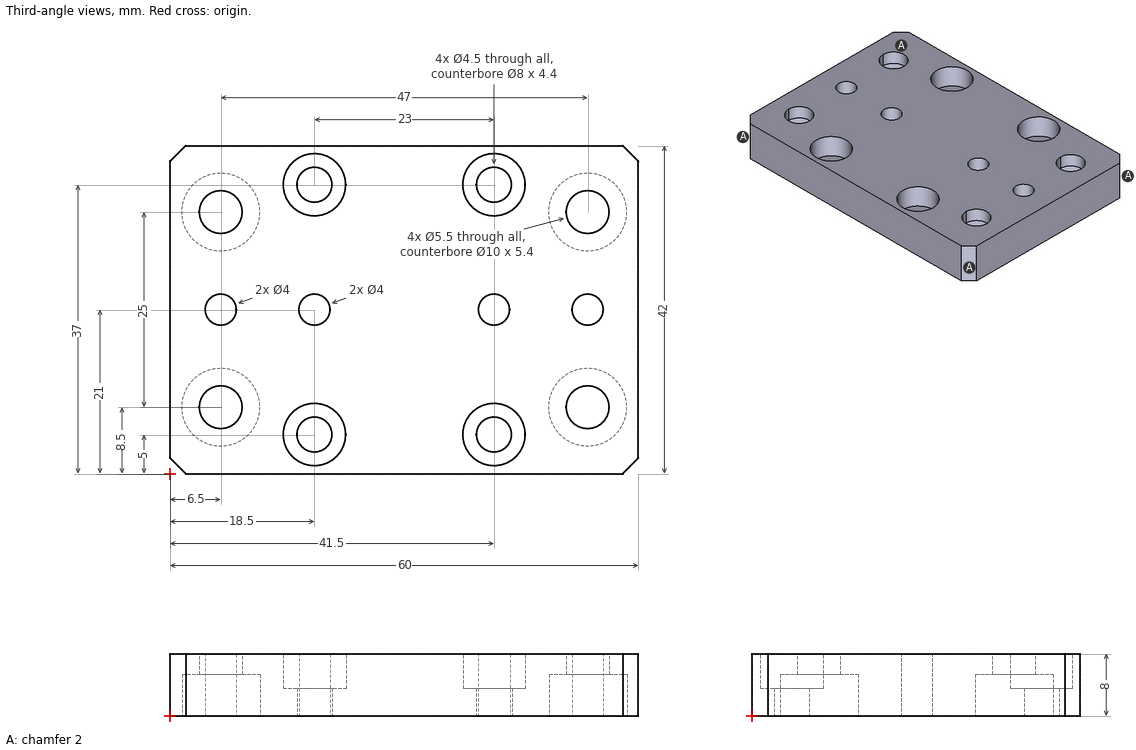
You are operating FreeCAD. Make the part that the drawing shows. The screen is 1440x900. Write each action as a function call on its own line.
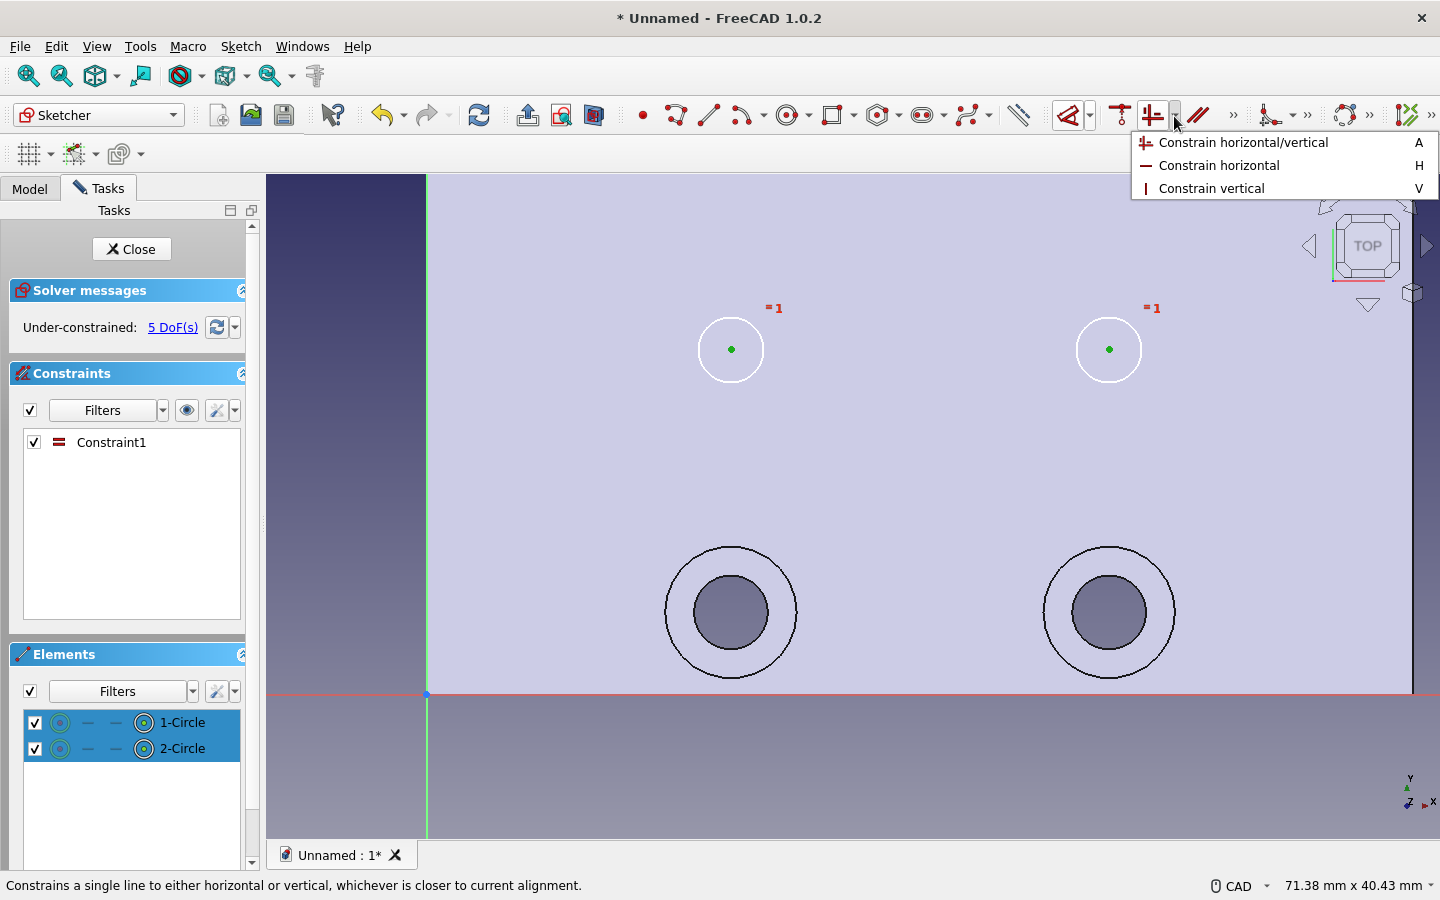
click(1285, 166)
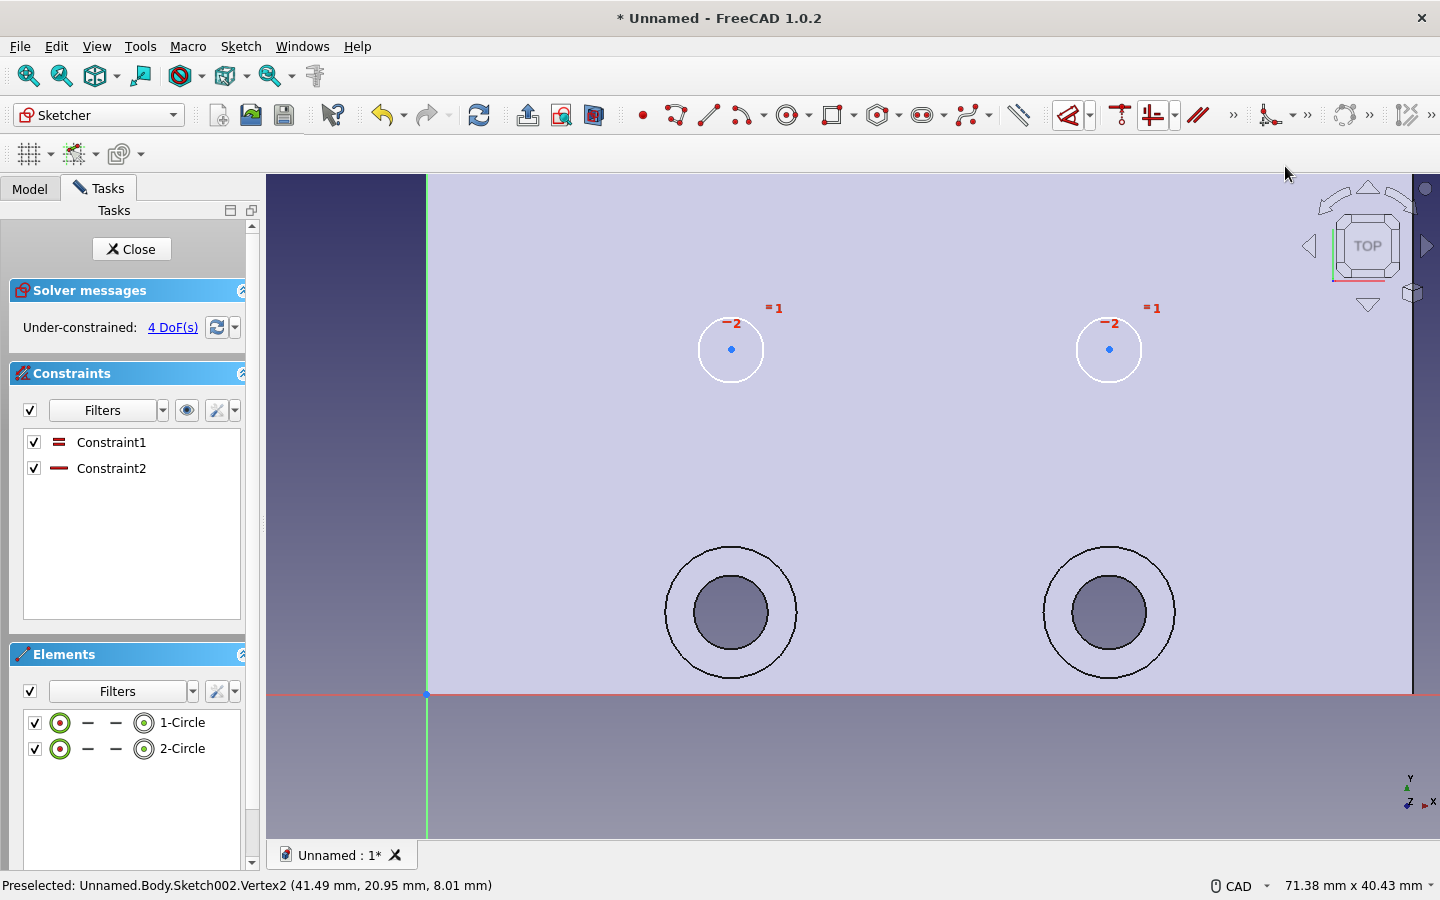
click(754, 327)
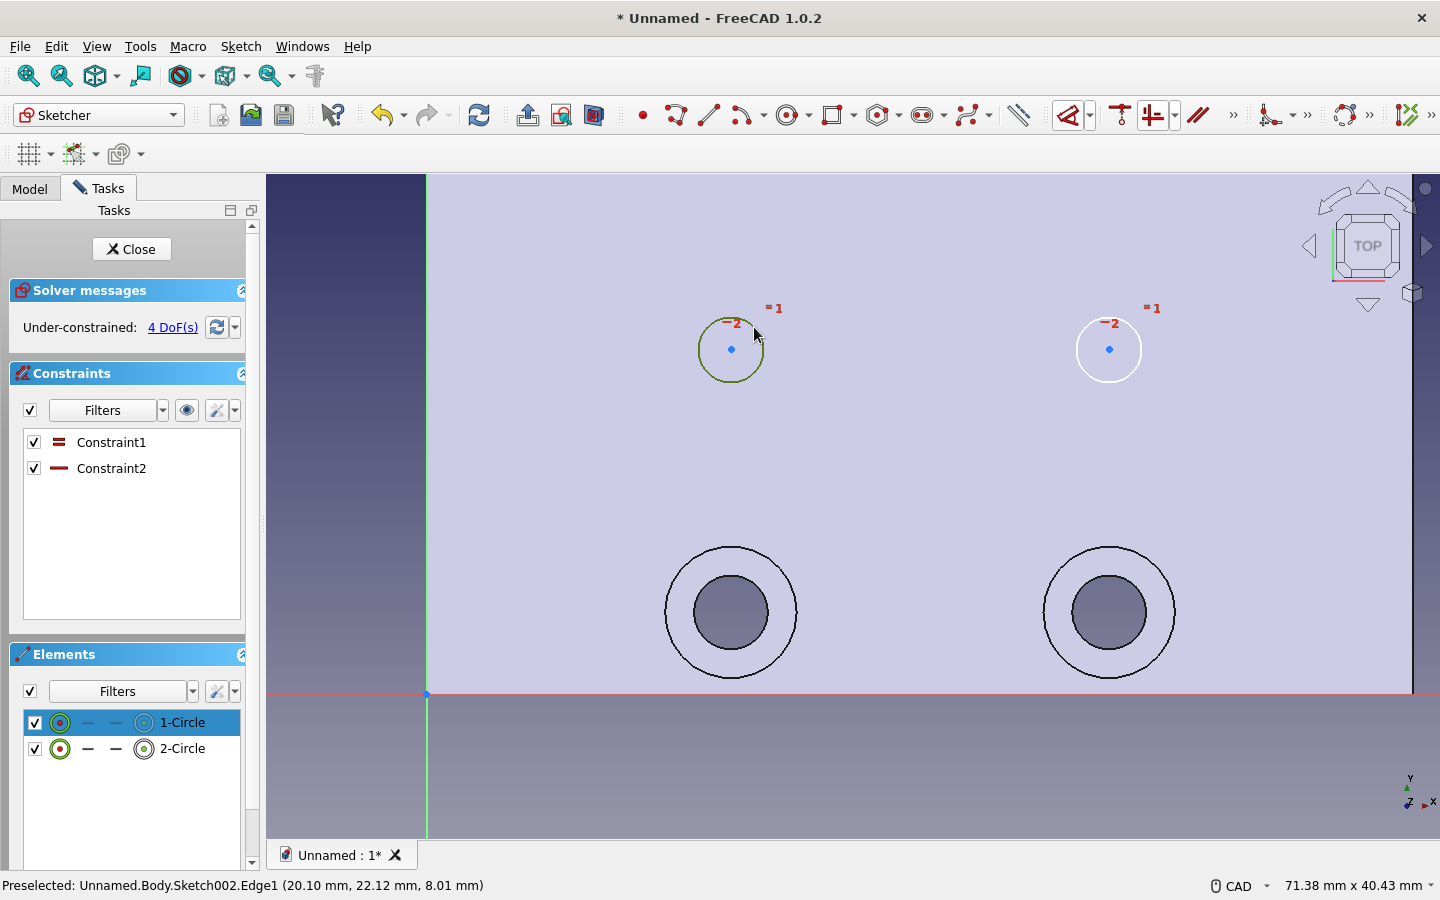
key(k)
key(o)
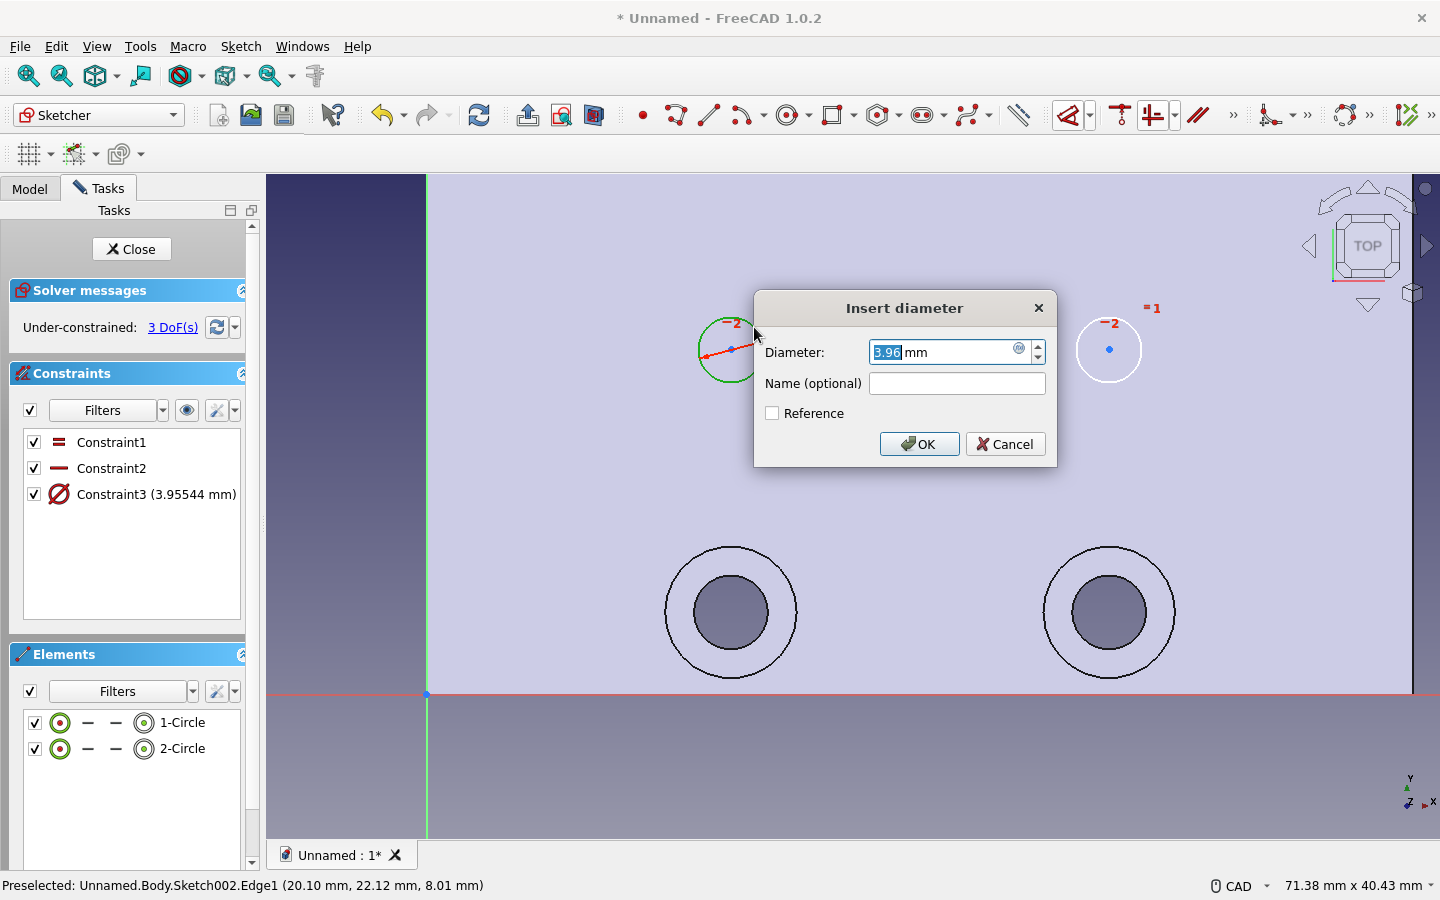
text(4)
key(Return)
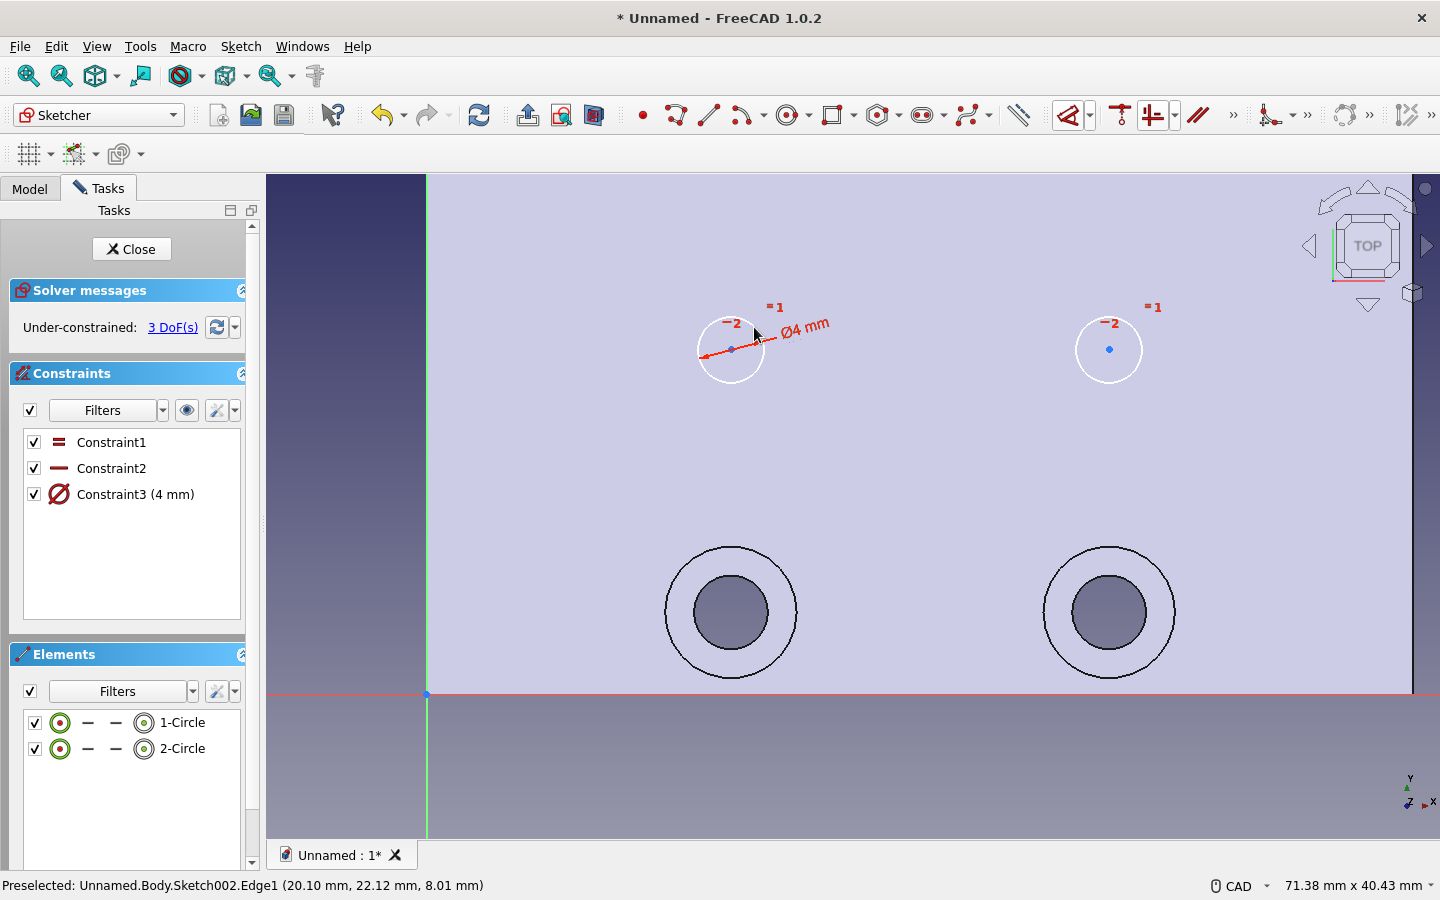
click(731, 350)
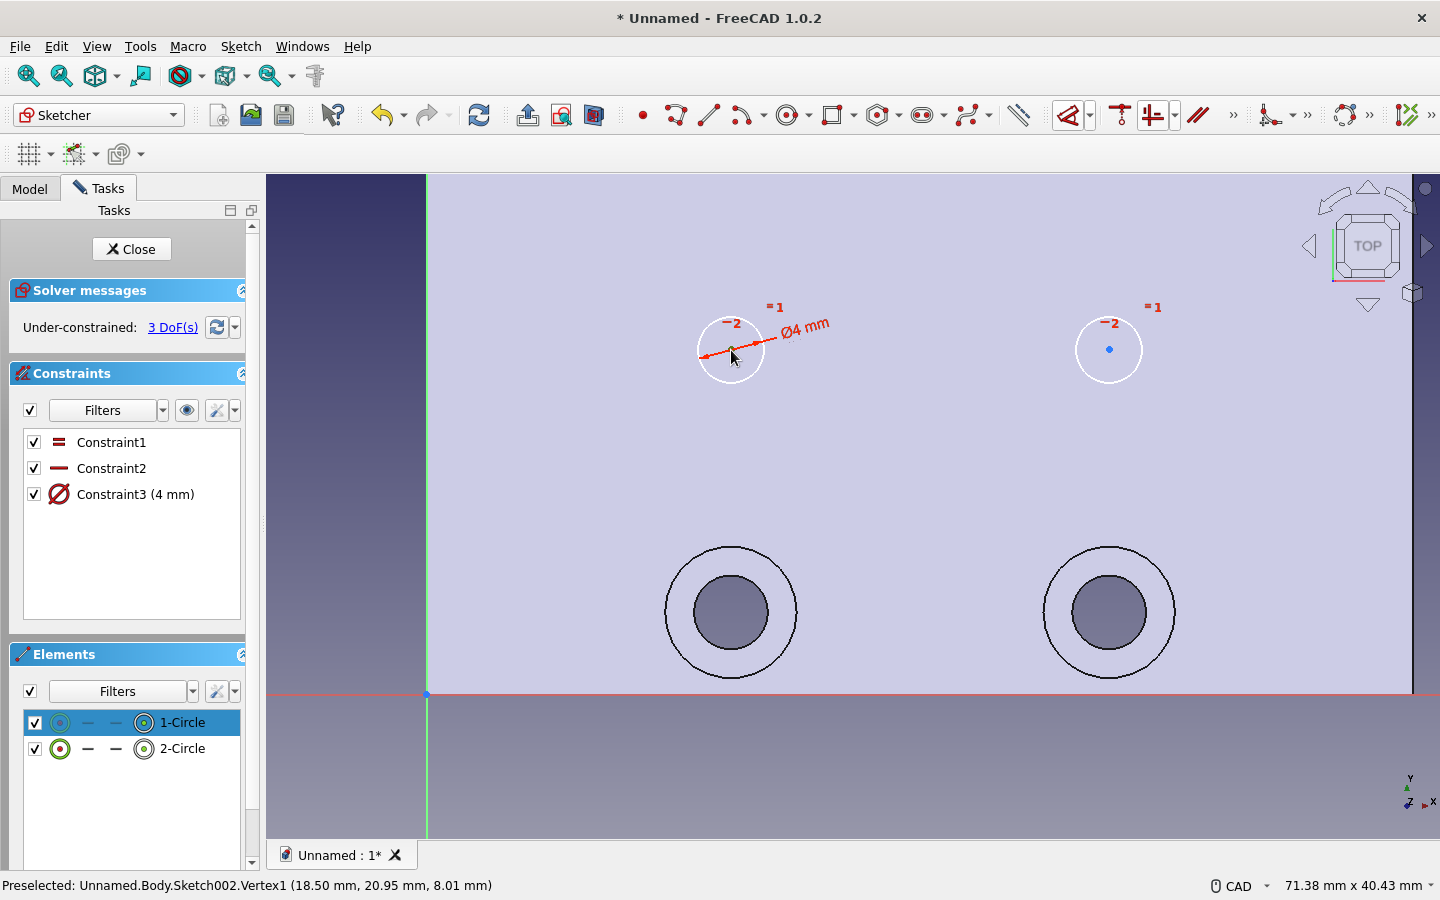
click(1090, 116)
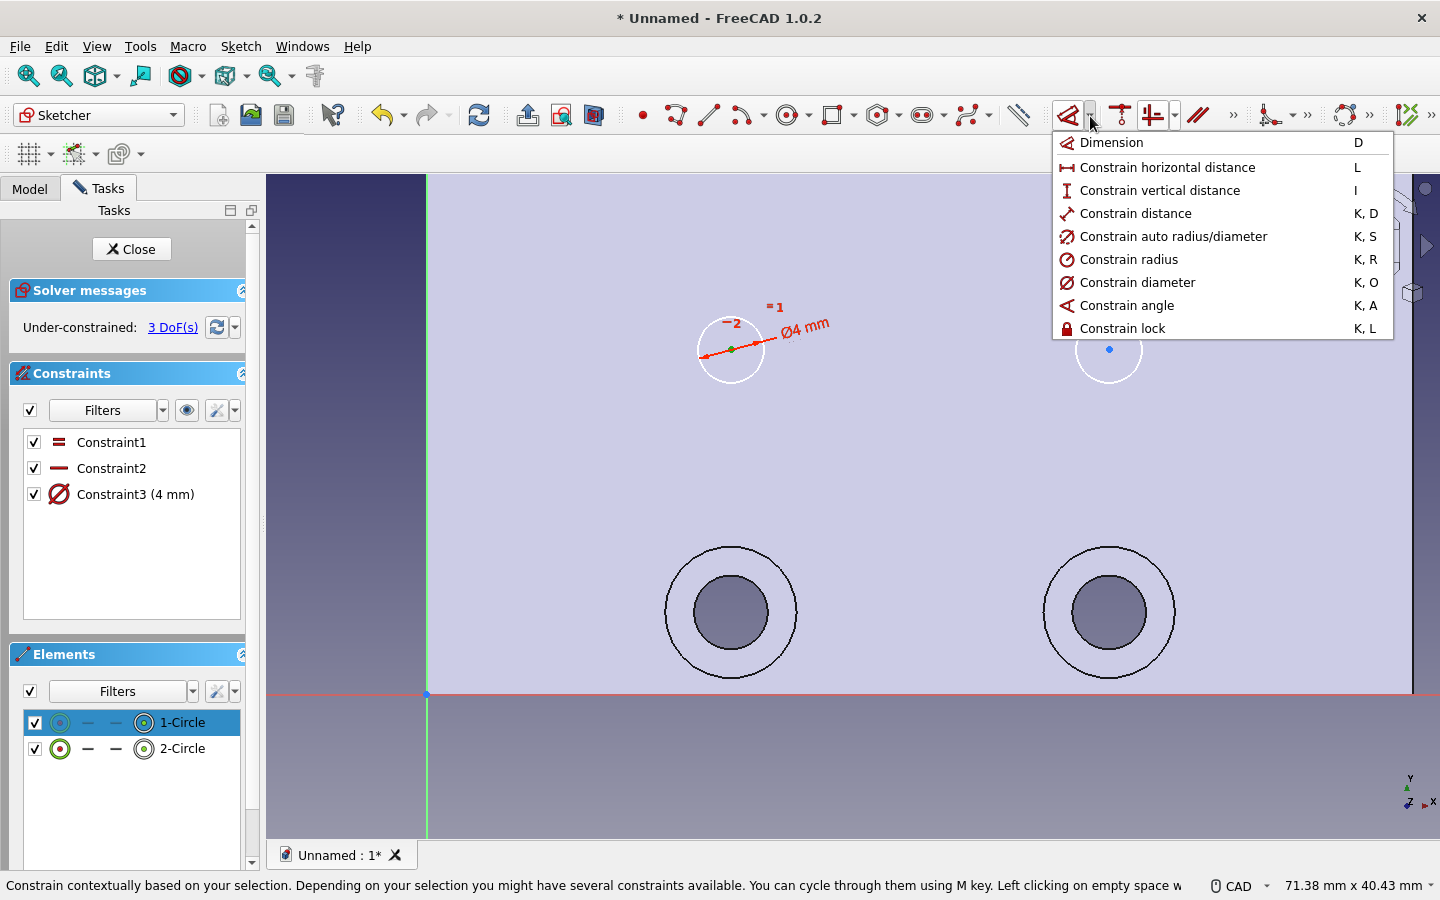
click(1223, 190)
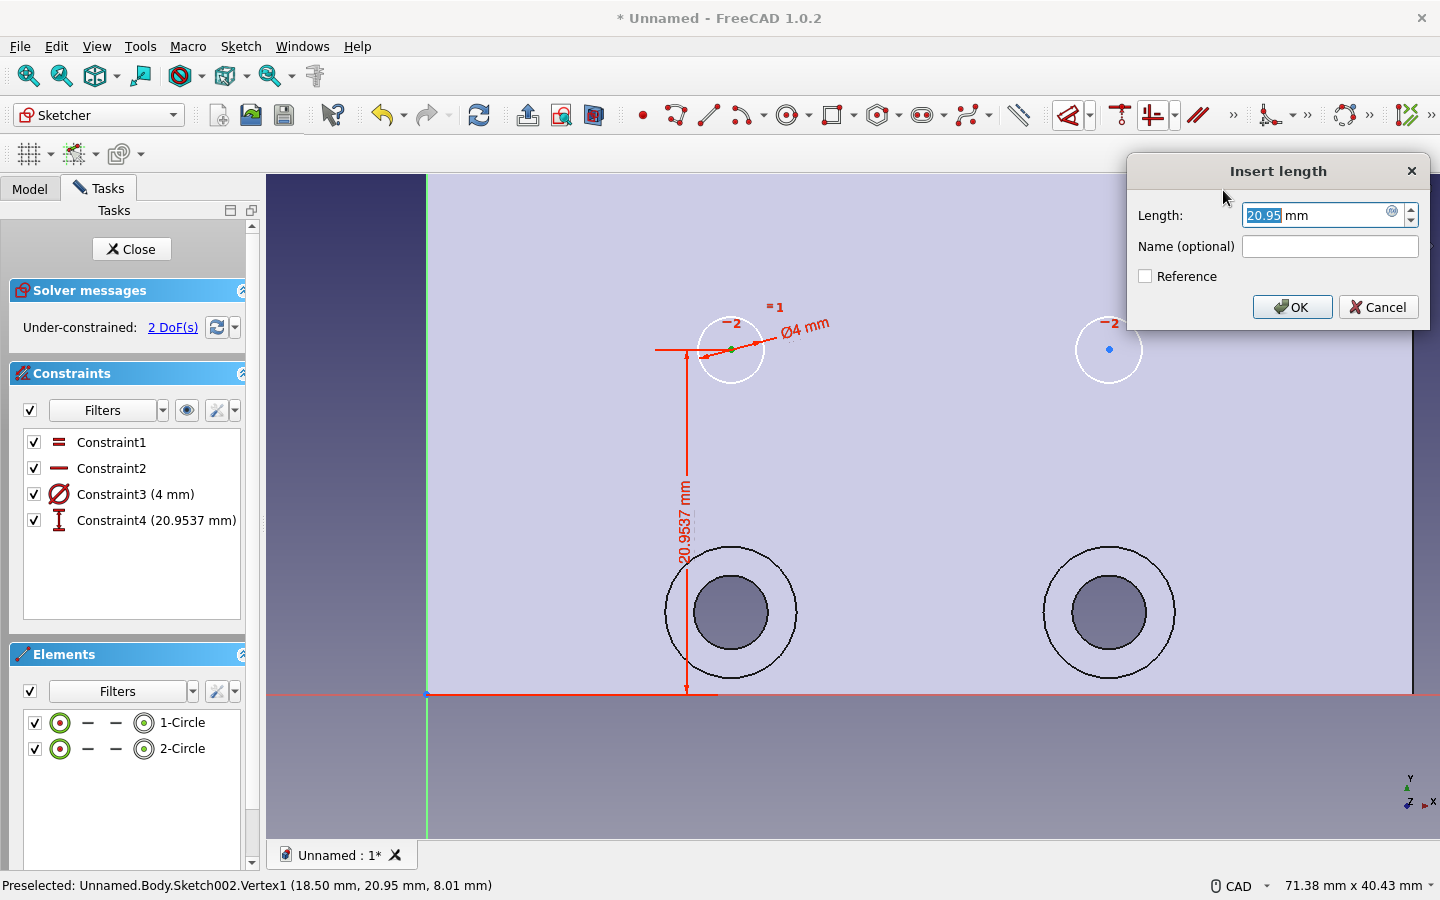
text(21)
key(Return)